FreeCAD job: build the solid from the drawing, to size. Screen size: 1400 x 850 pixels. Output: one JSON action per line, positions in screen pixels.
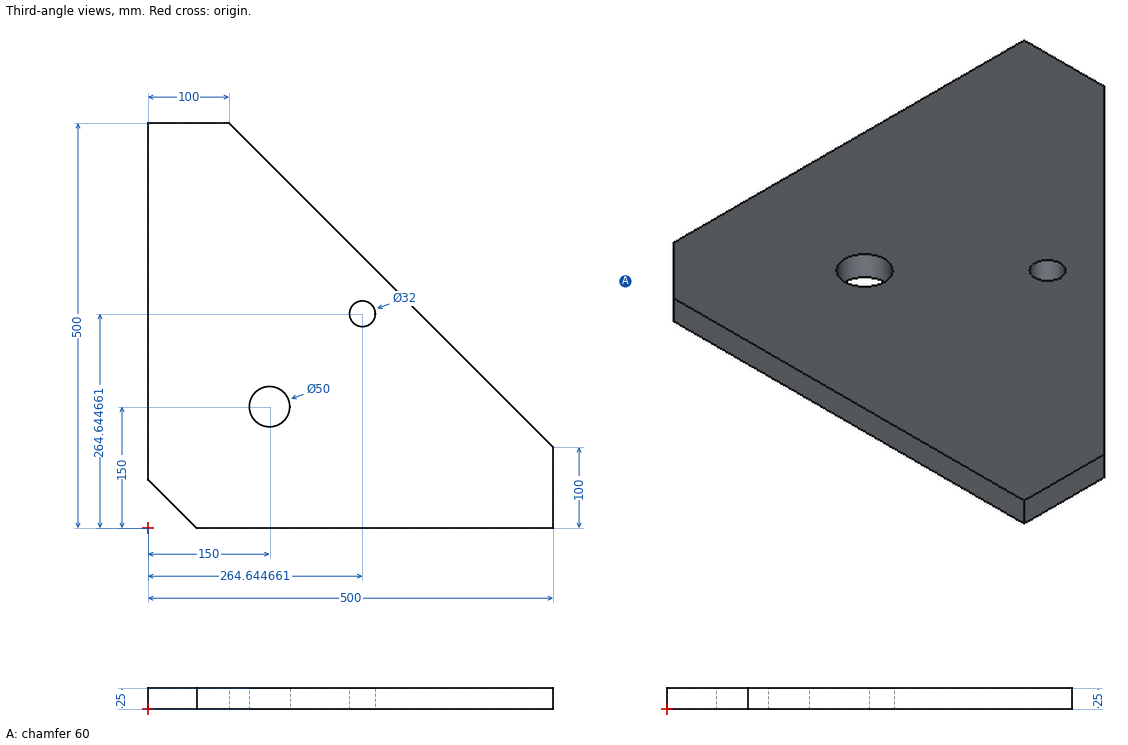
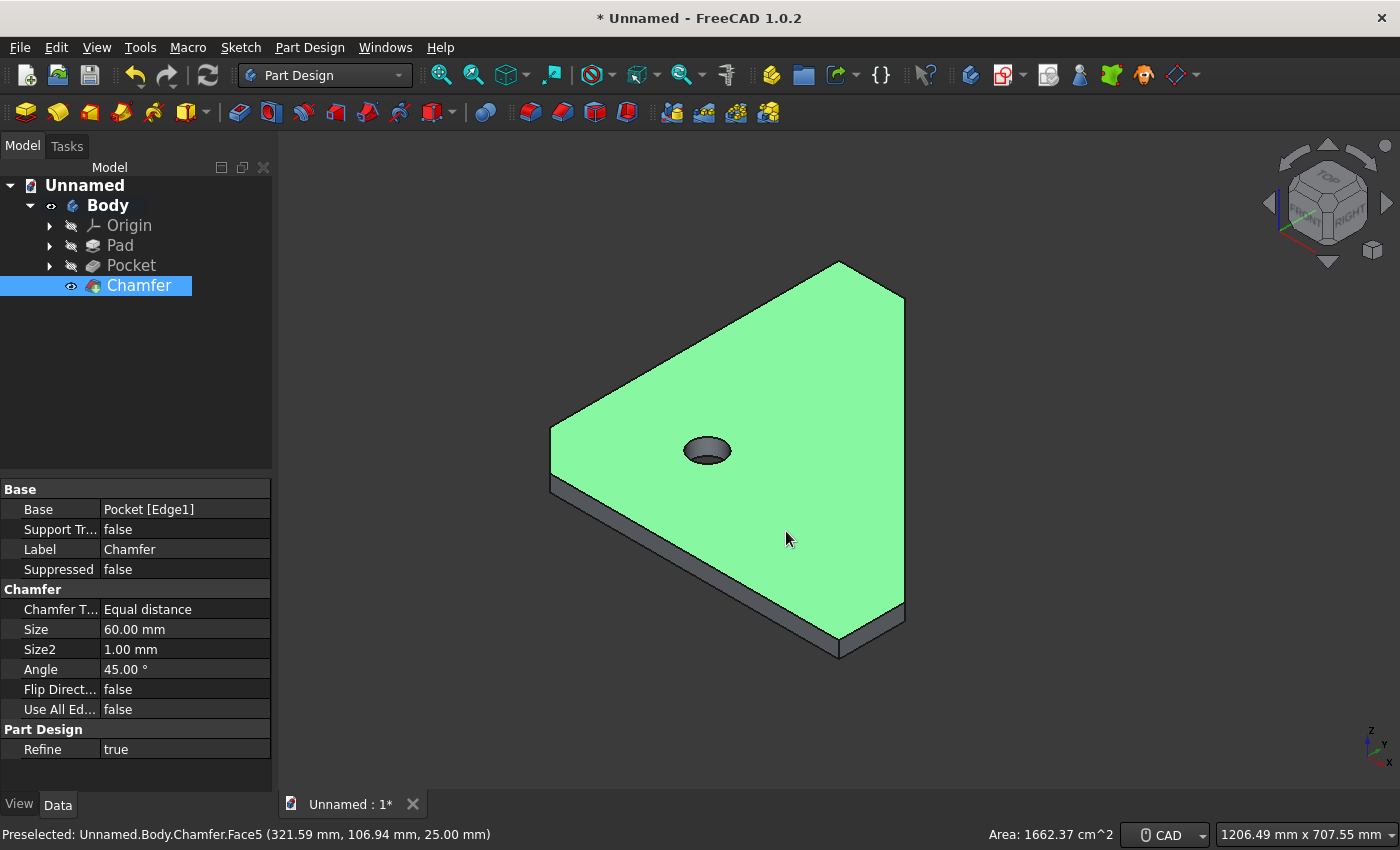
{"action": "left_click", "coordinate": [1004, 76]}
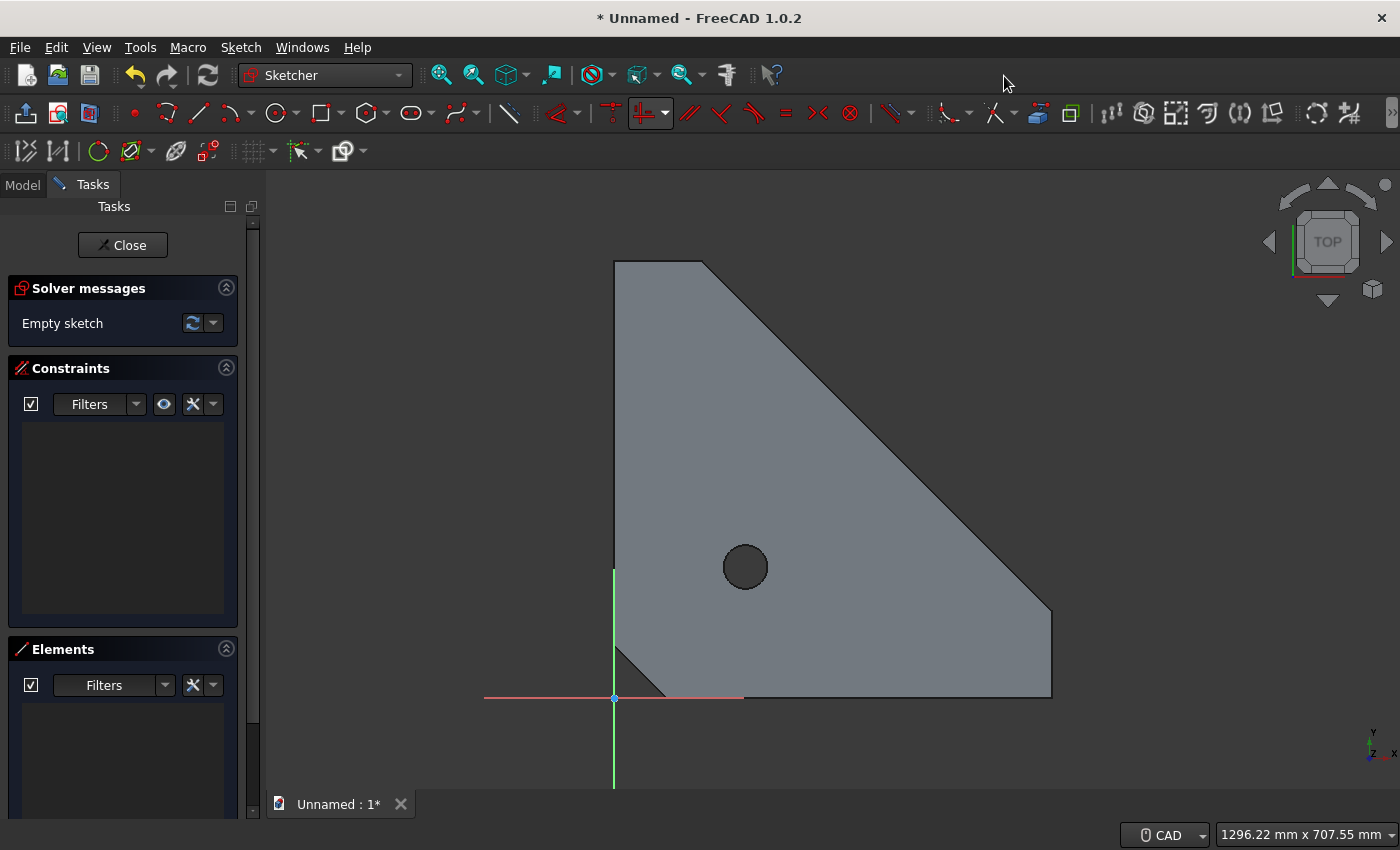
{"action": "scroll", "coordinate": [852, 466], "scroll_direction": "up", "scroll_amount": 13}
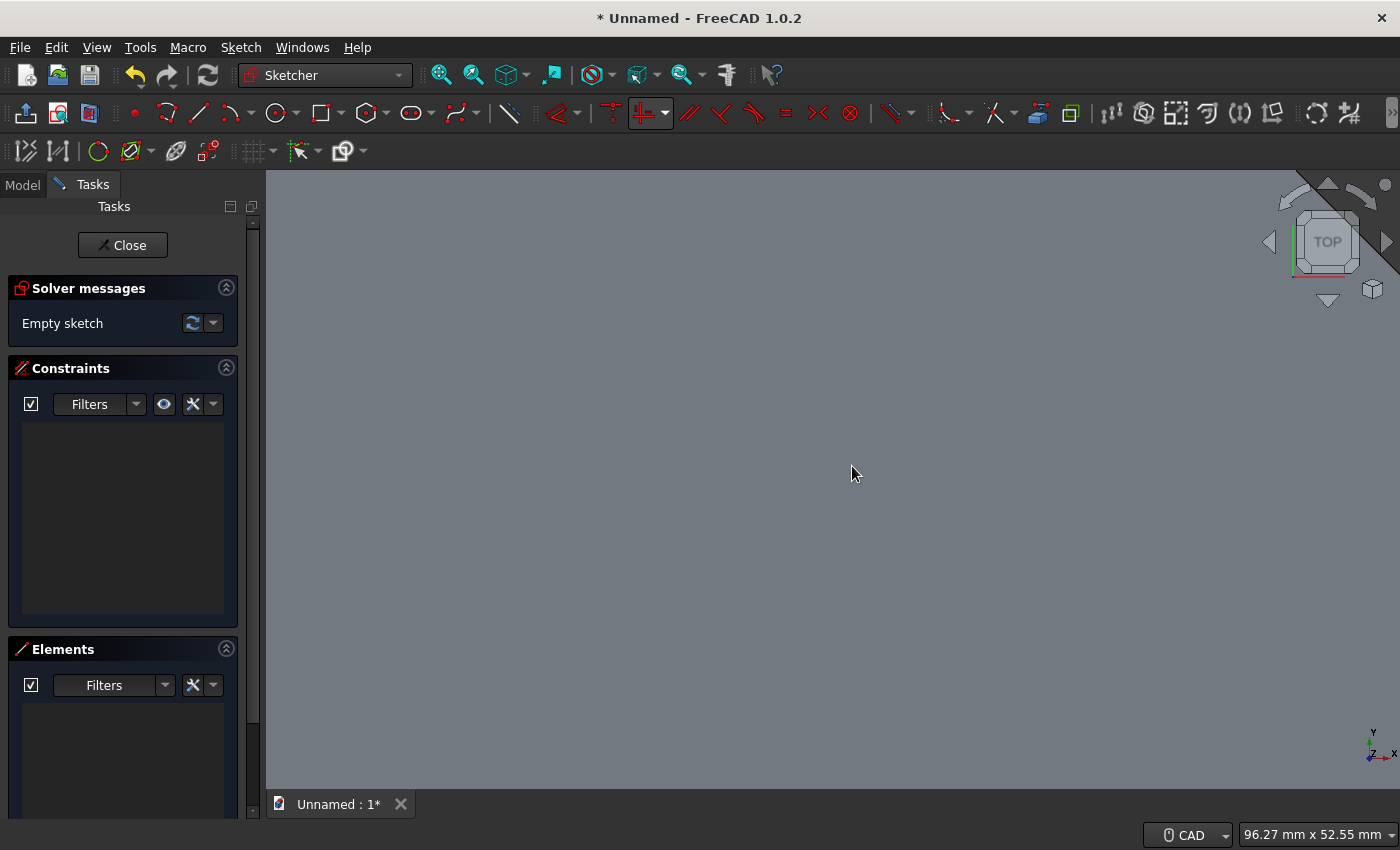
{"action": "left_click", "coordinate": [276, 114]}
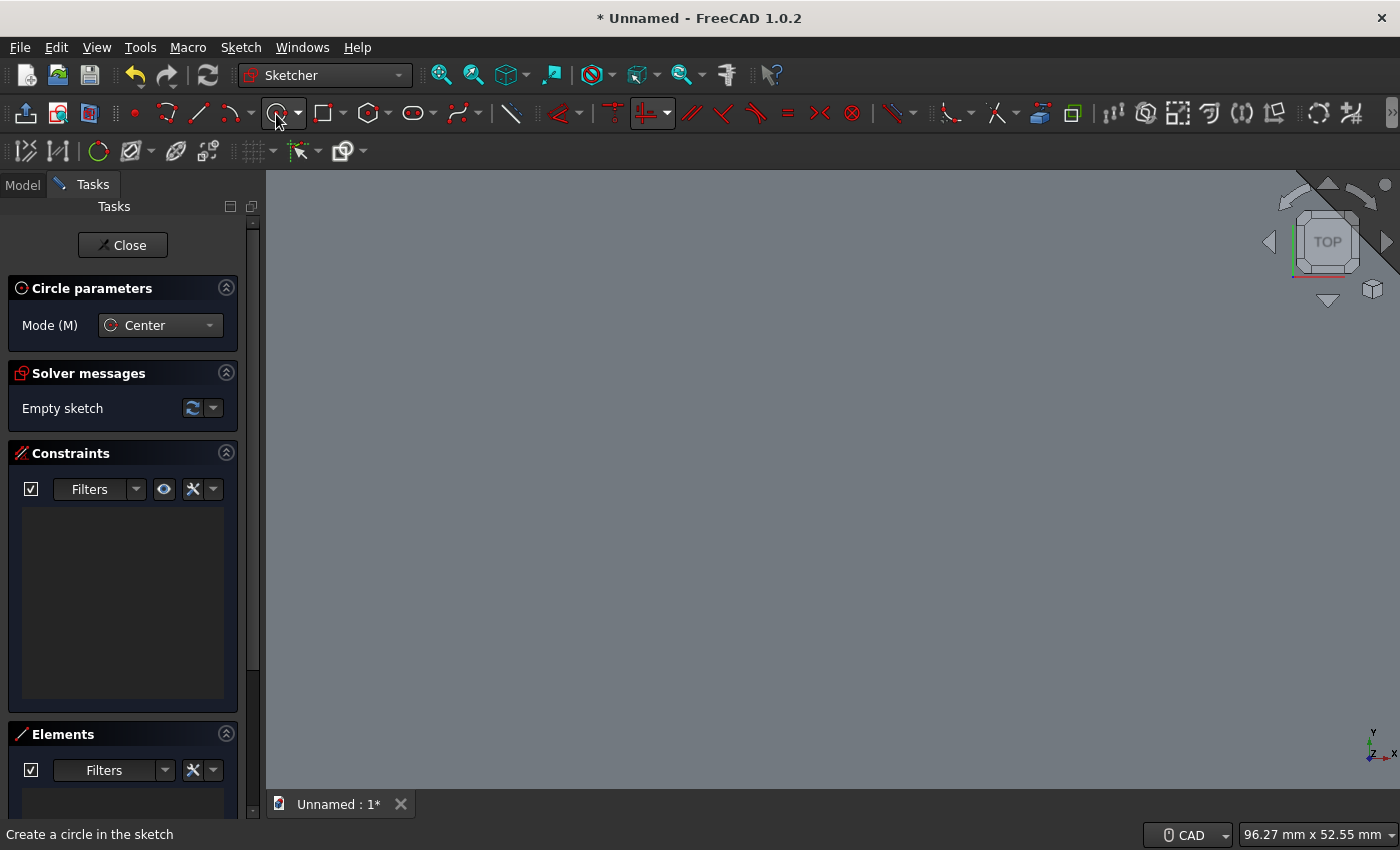
{"action": "left_click", "coordinate": [762, 469]}
{"action": "left_click", "coordinate": [896, 336]}
{"action": "key", "text": "Escape"}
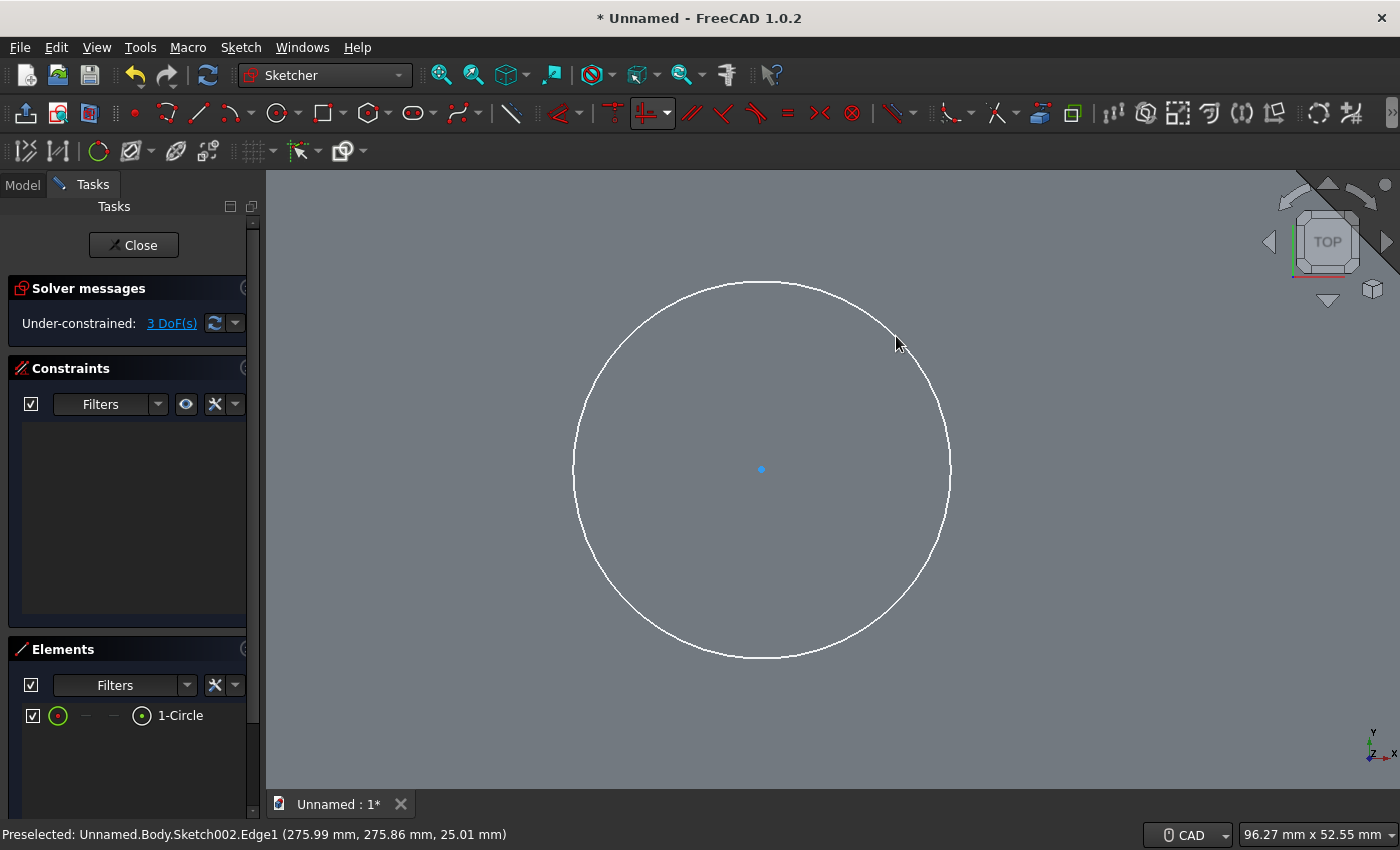
{"action": "left_click", "coordinate": [558, 114]}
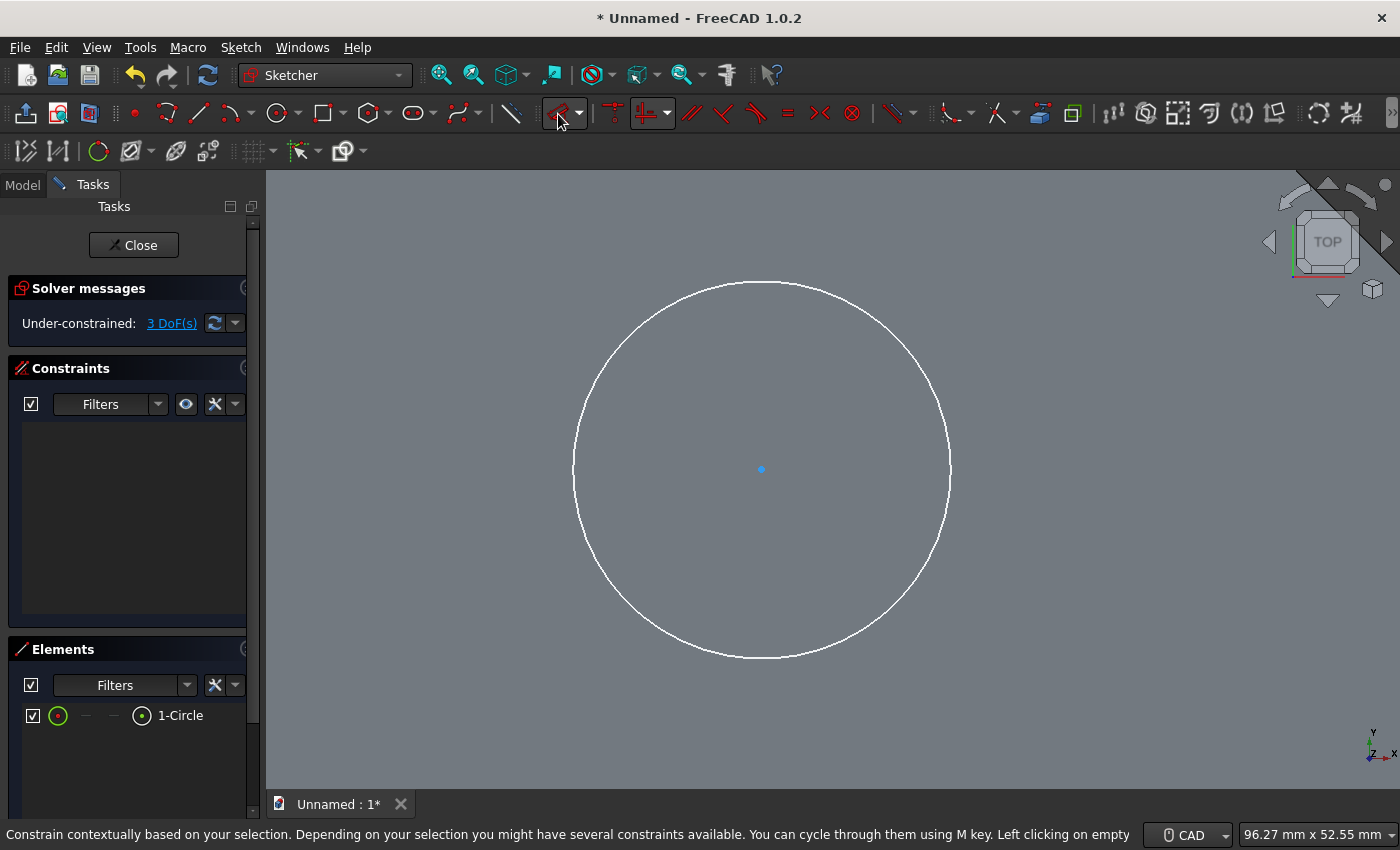
{"action": "left_click", "coordinate": [895, 336]}
{"action": "left_click", "coordinate": [918, 313]}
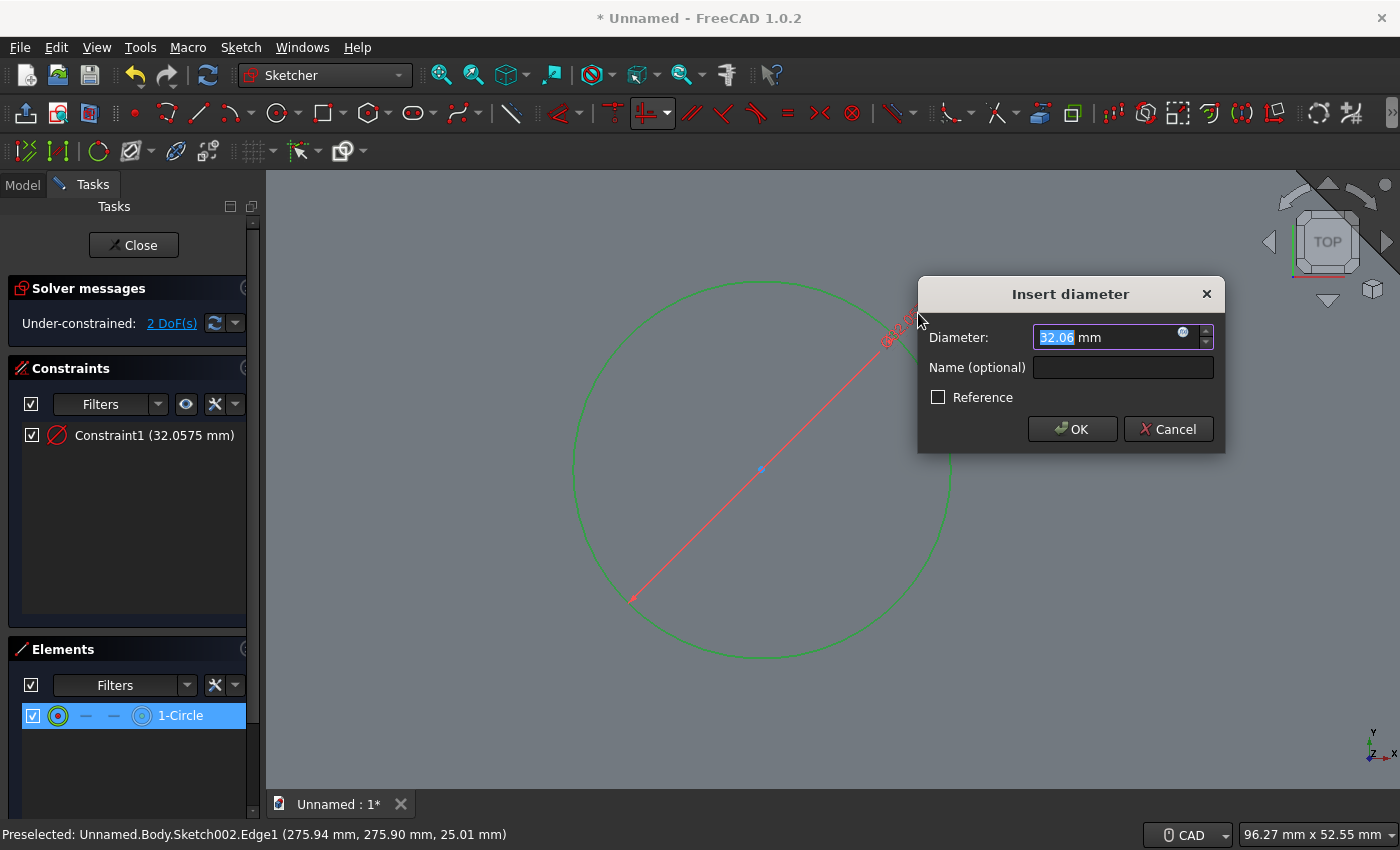
{"action": "type", "text": "32"}
{"action": "key", "text": "Return"}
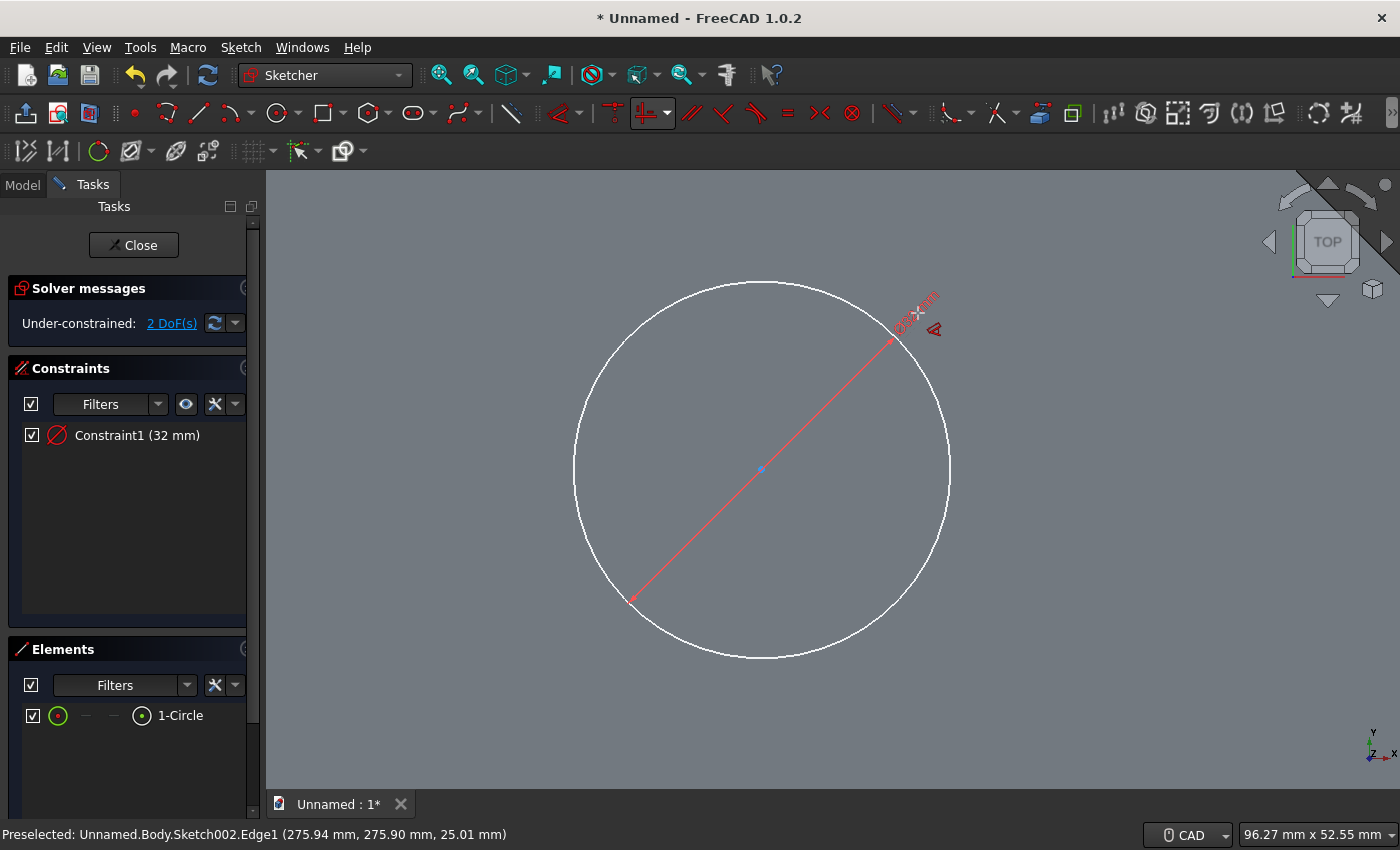
{"action": "left_click", "coordinate": [762, 470]}
{"action": "left_click", "coordinate": [528, 436]}